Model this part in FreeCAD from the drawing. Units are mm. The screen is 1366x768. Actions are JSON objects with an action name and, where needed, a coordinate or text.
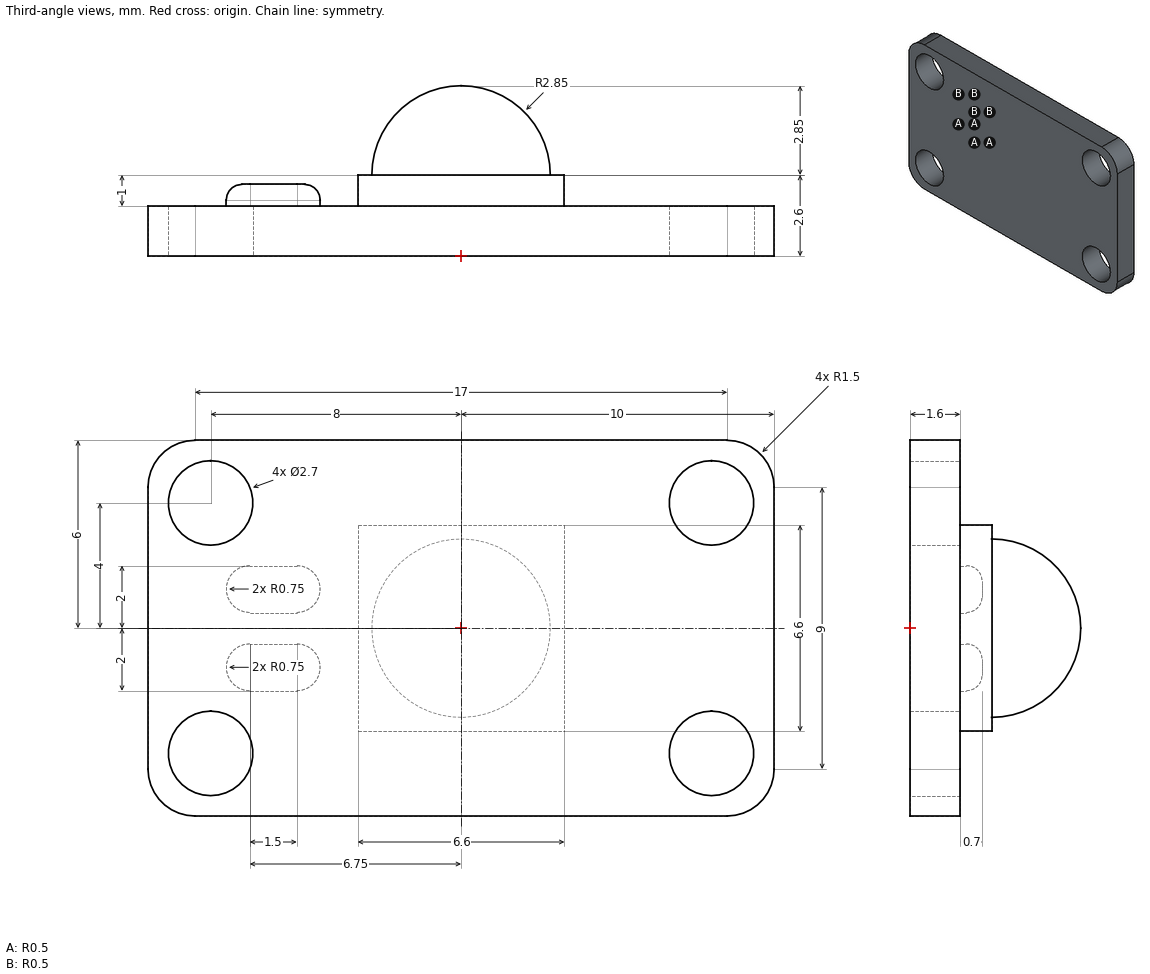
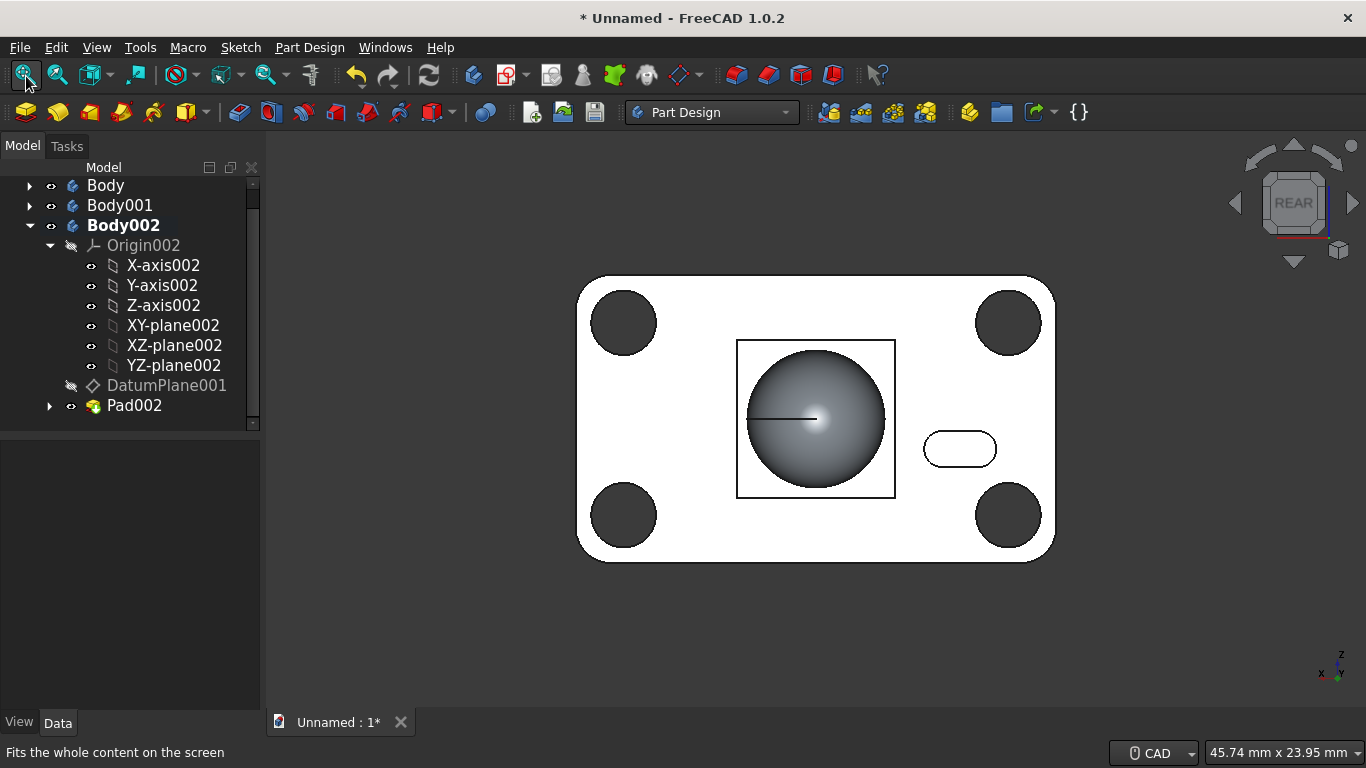
{"action": "left_click", "coordinate": [26, 76]}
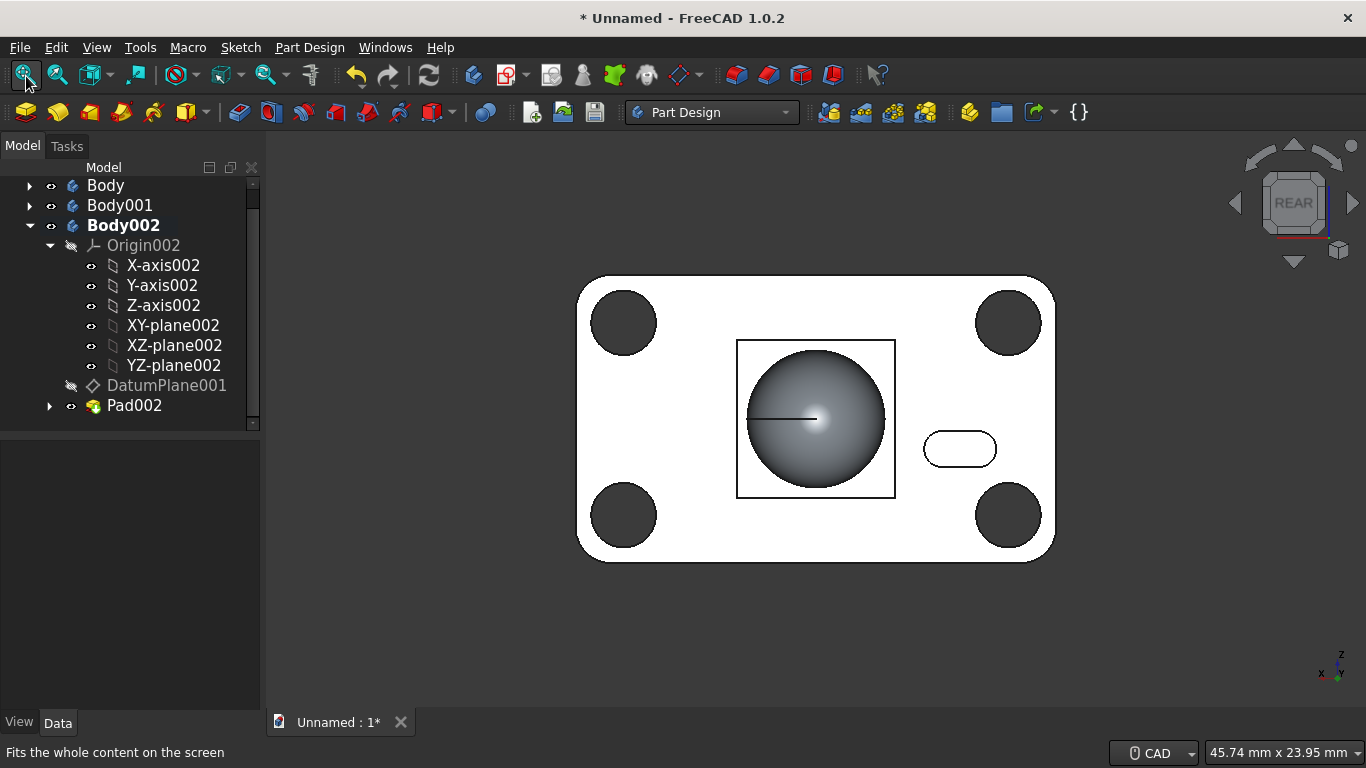
{"action": "left_click", "coordinate": [950, 448]}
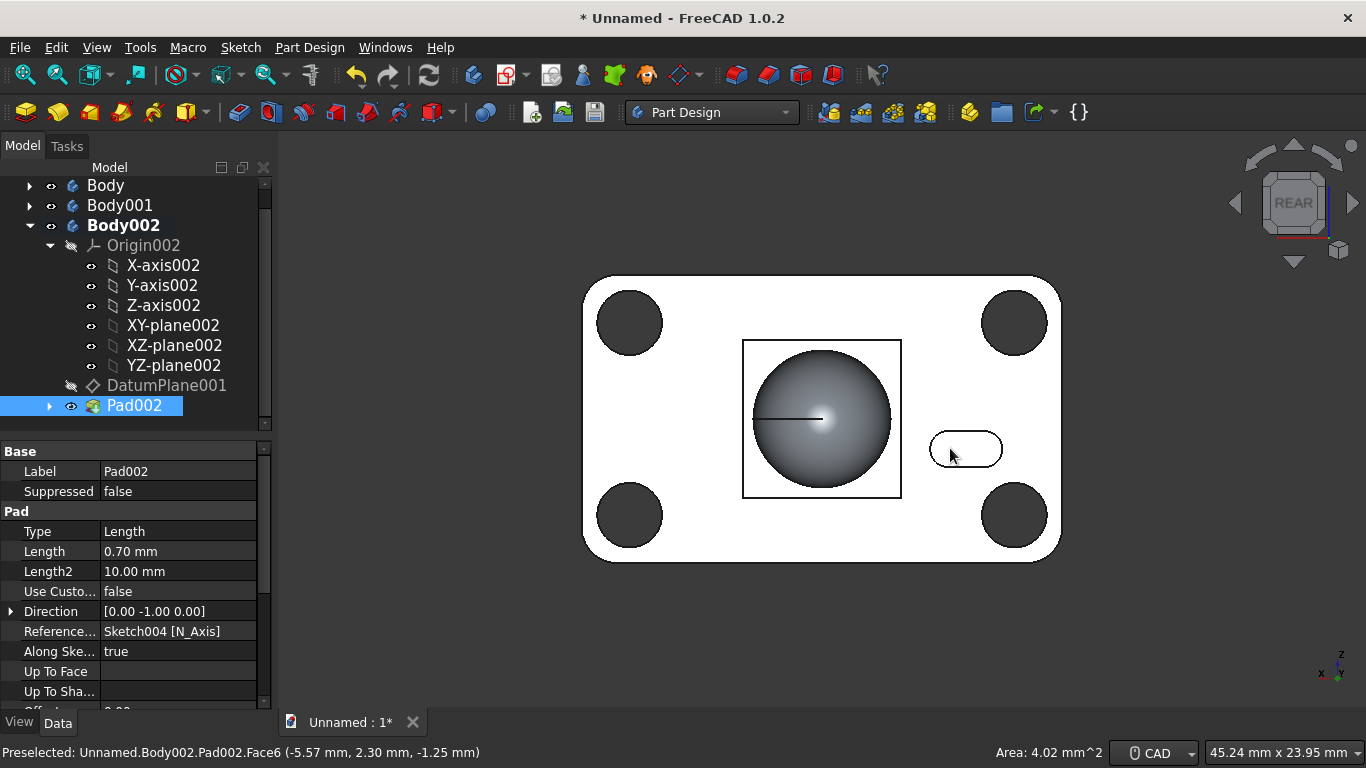
{"action": "left_click", "coordinate": [738, 76]}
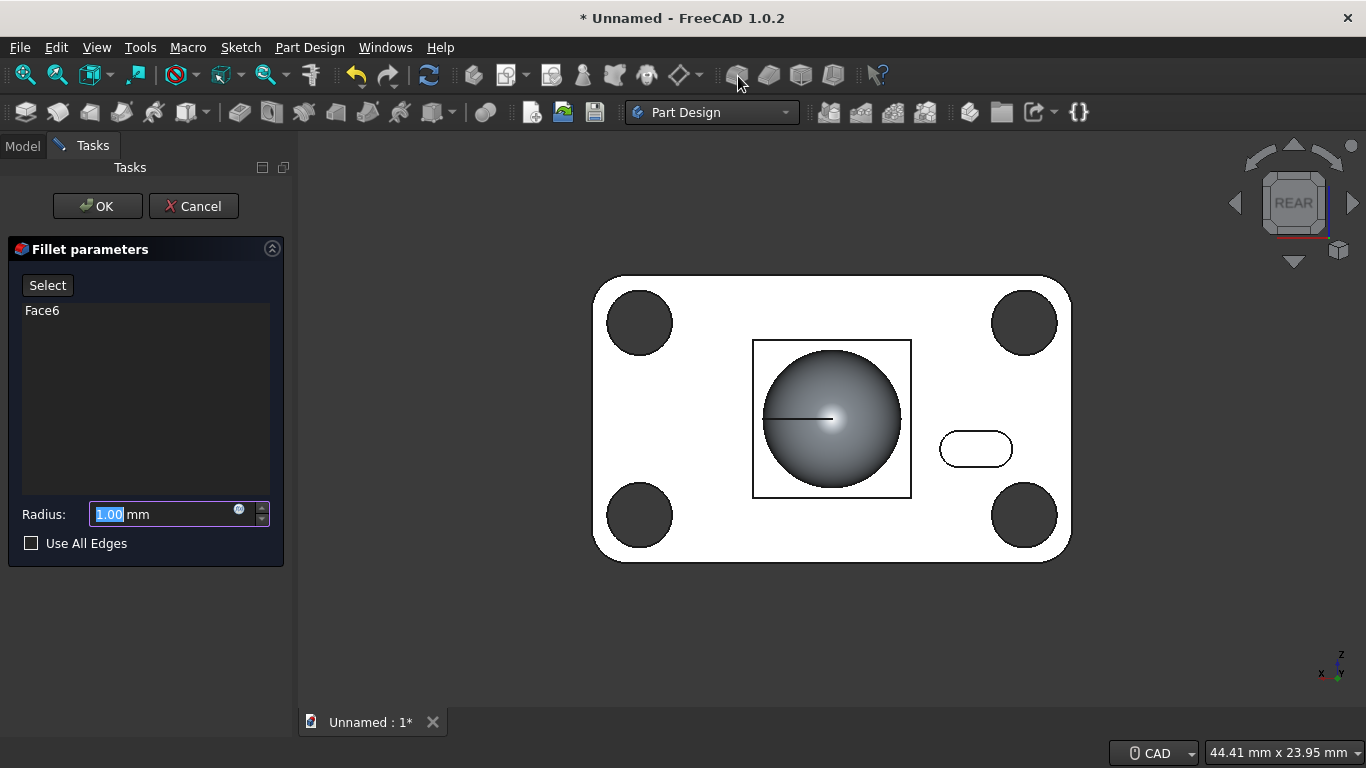
{"action": "type", "text": "0.5"}
{"action": "key", "text": "Tab"}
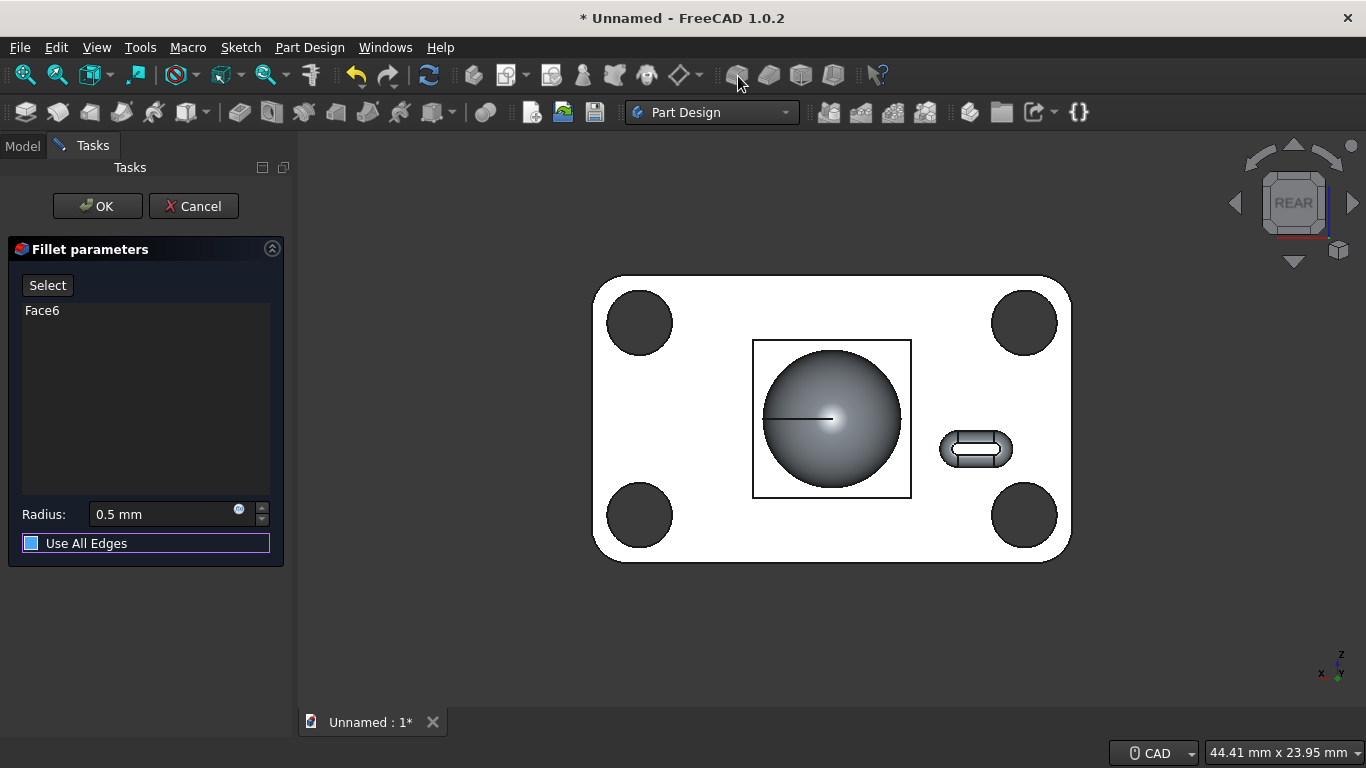
{"action": "left_click", "coordinate": [98, 206]}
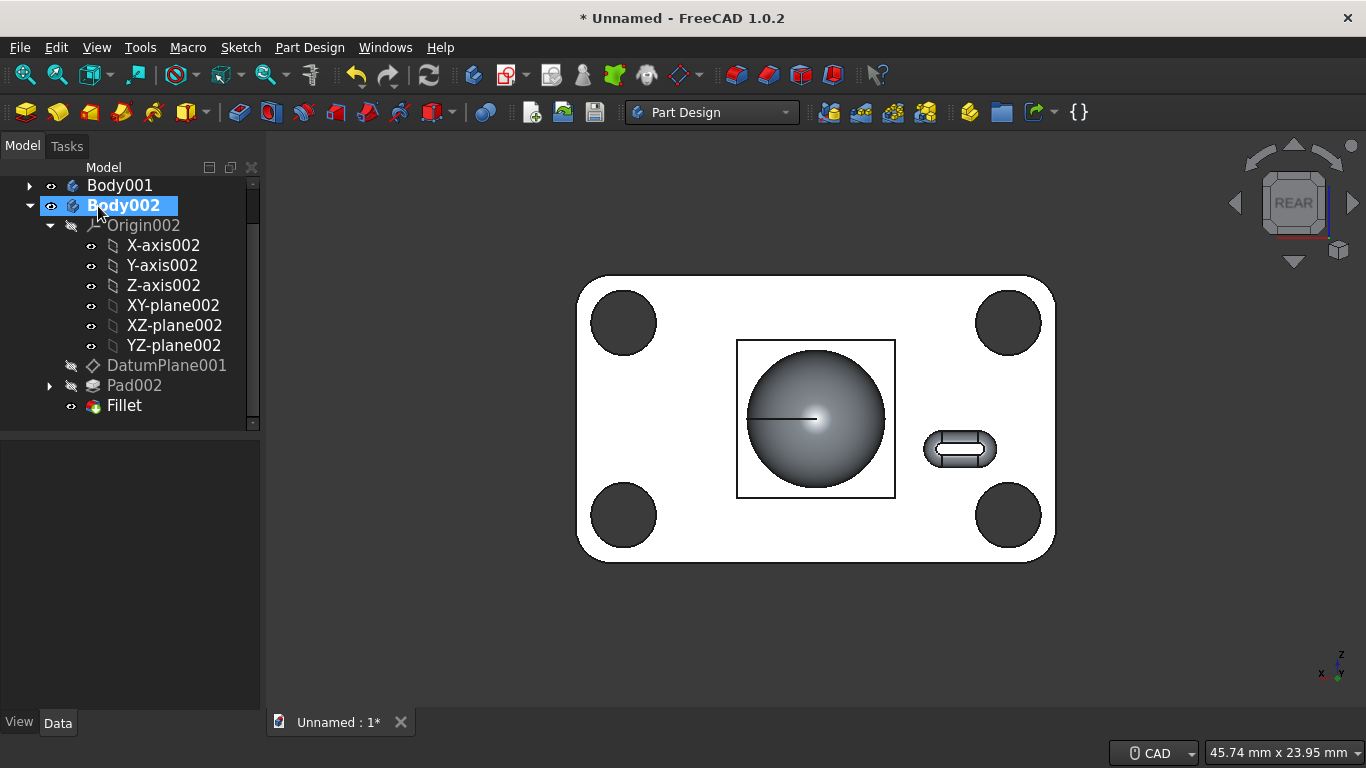
{"action": "left_click", "coordinate": [26, 76]}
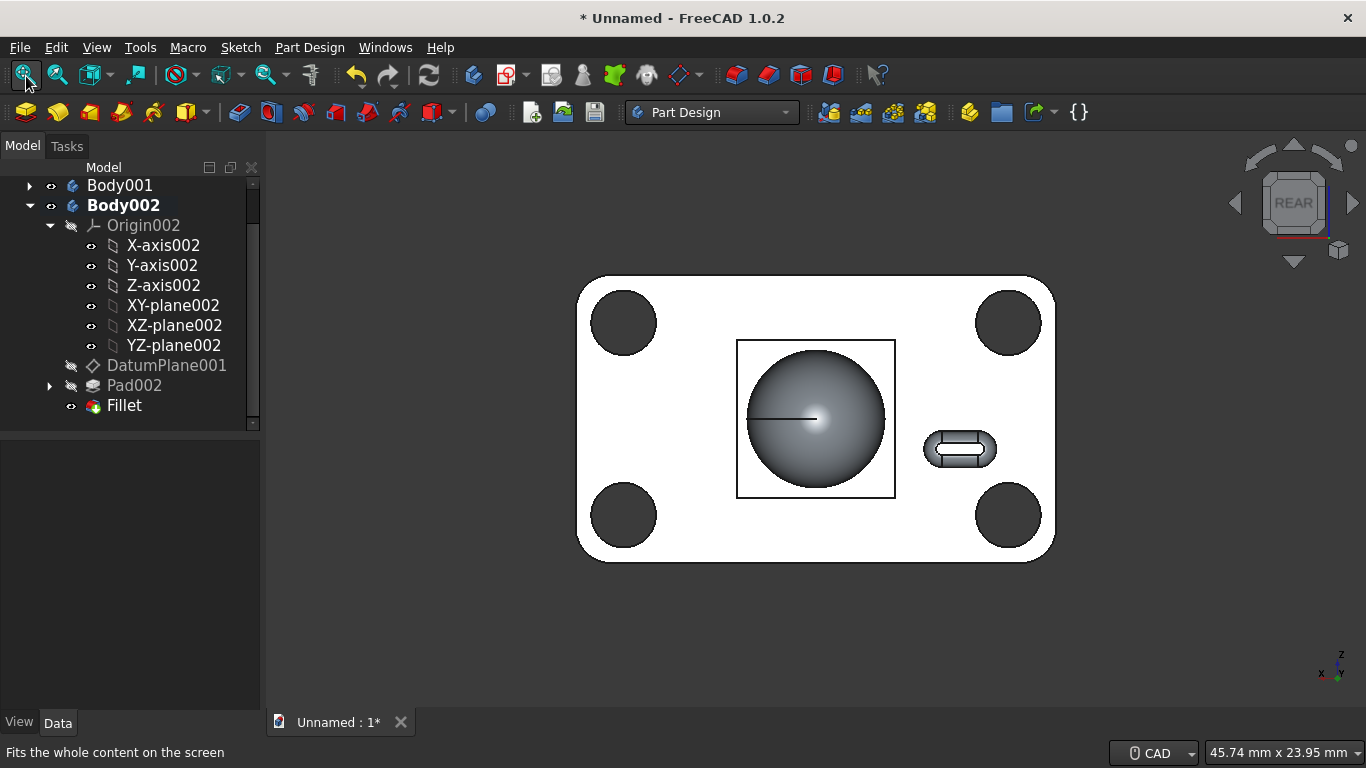
{"action": "left_click", "coordinate": [474, 76]}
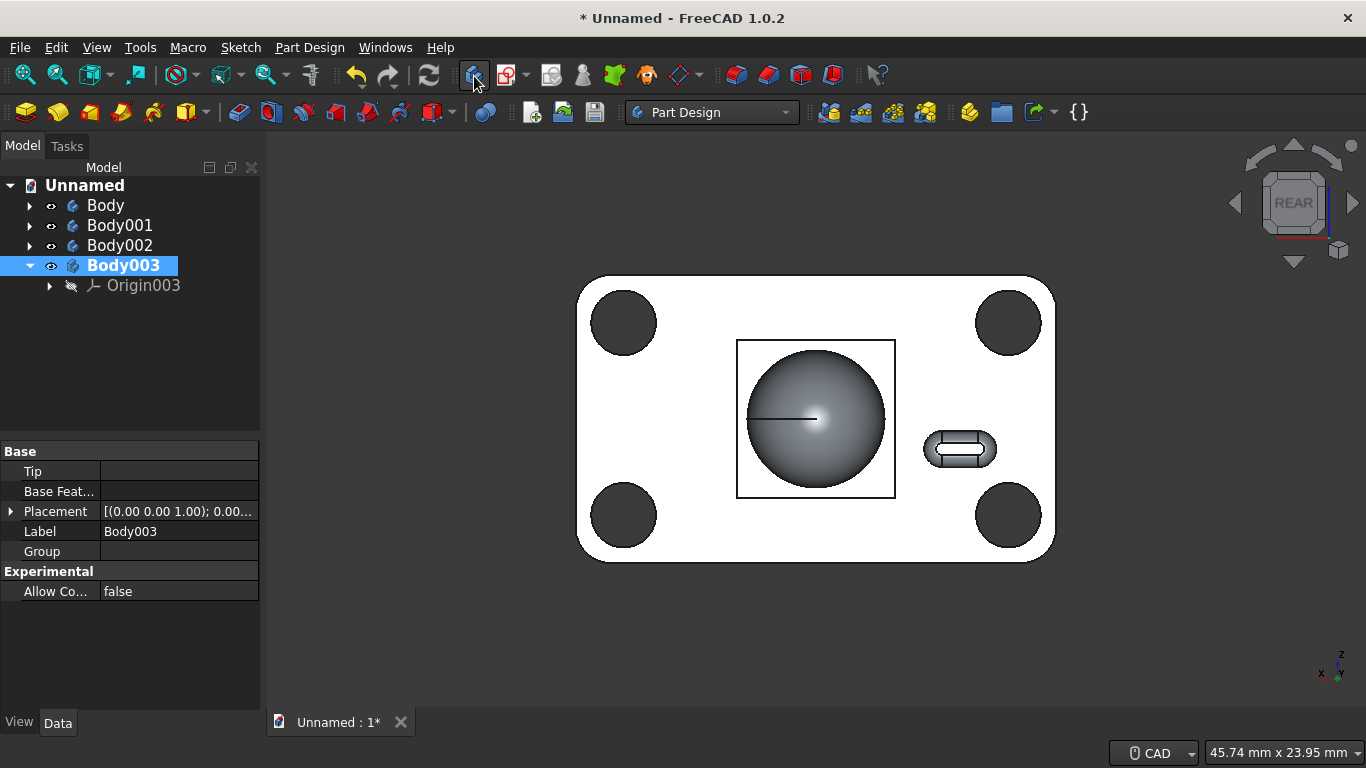
{"action": "left_click", "coordinate": [50, 286]}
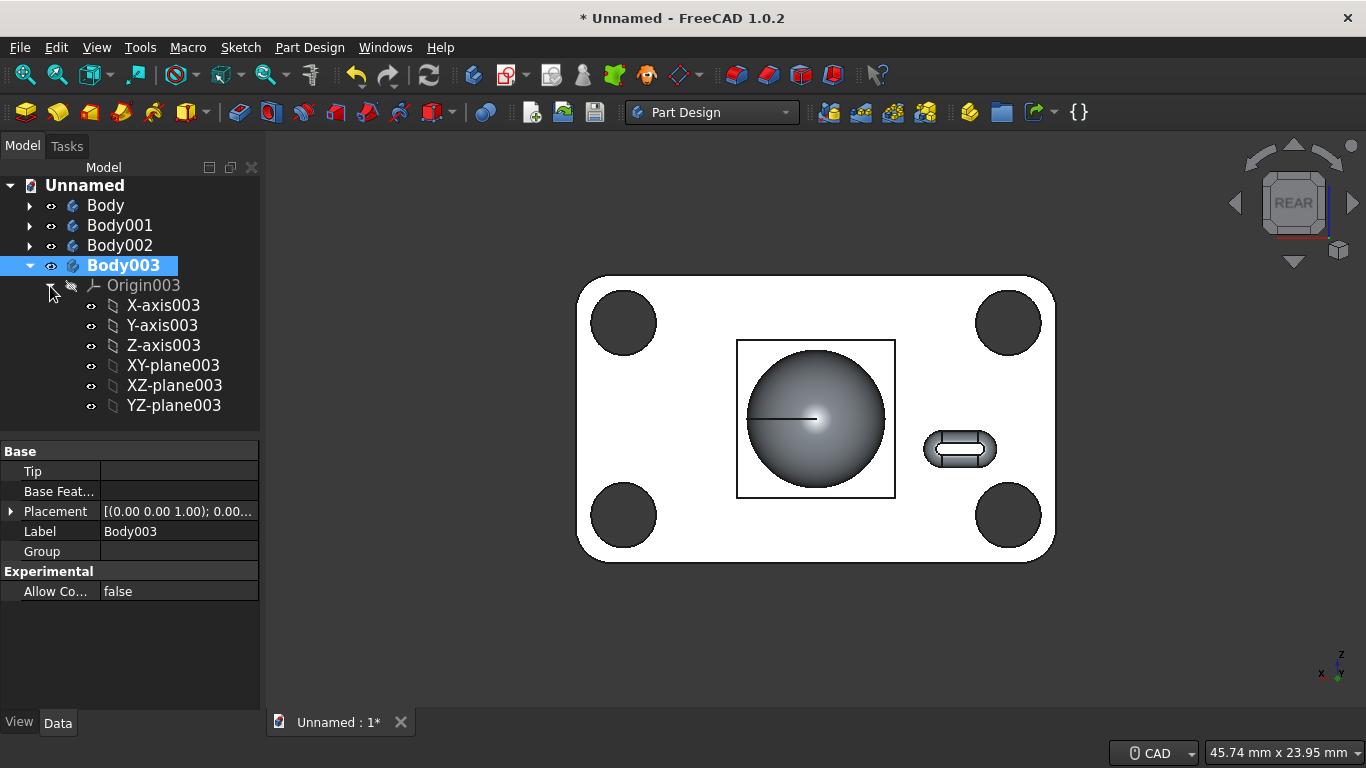
{"action": "left_click", "coordinate": [136, 386]}